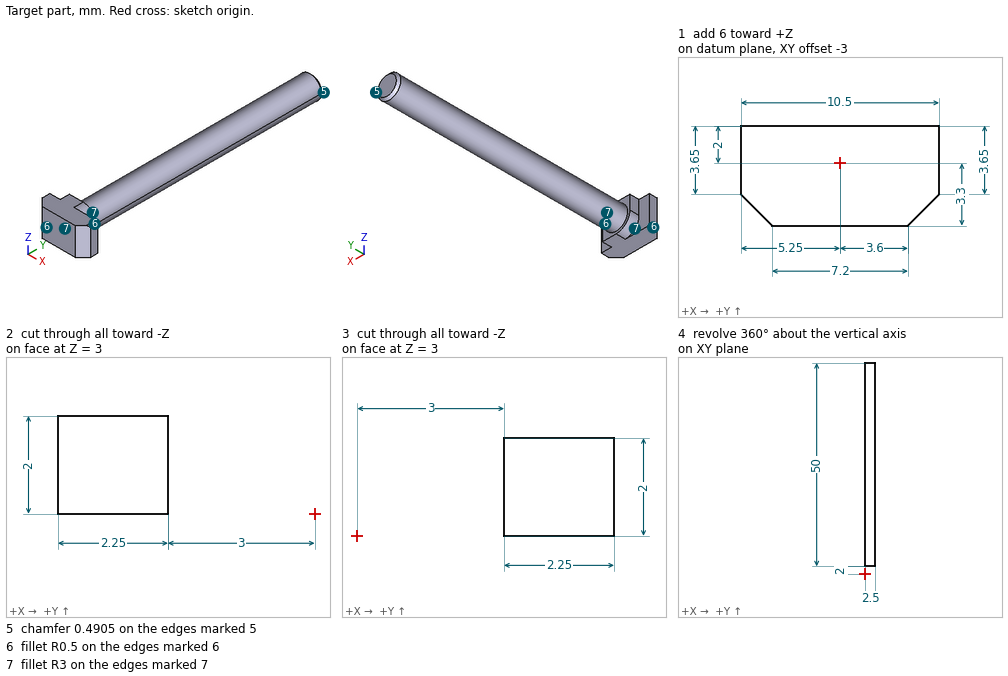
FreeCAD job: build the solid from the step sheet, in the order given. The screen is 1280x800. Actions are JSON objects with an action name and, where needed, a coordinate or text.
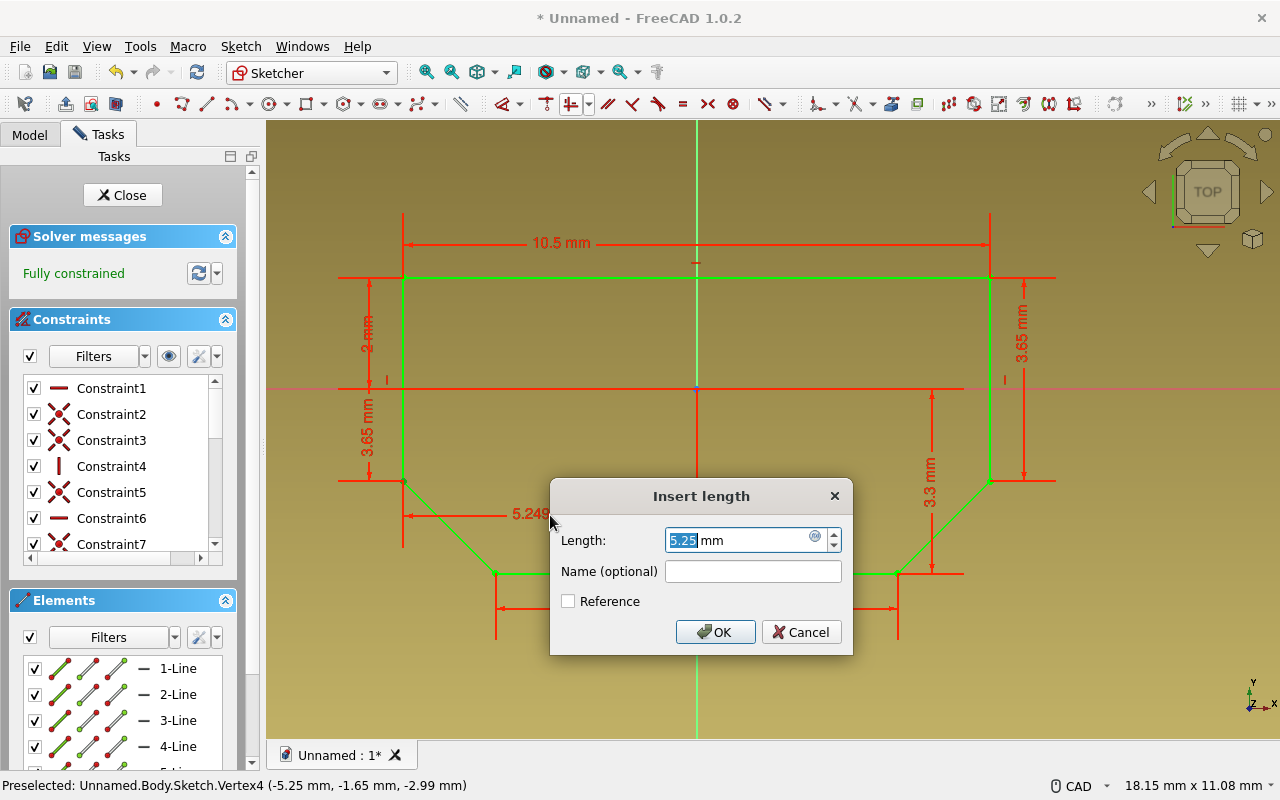
{"action": "type", "text": "5.25"}
{"action": "key", "text": "Return"}
{"action": "key", "text": "Escape"}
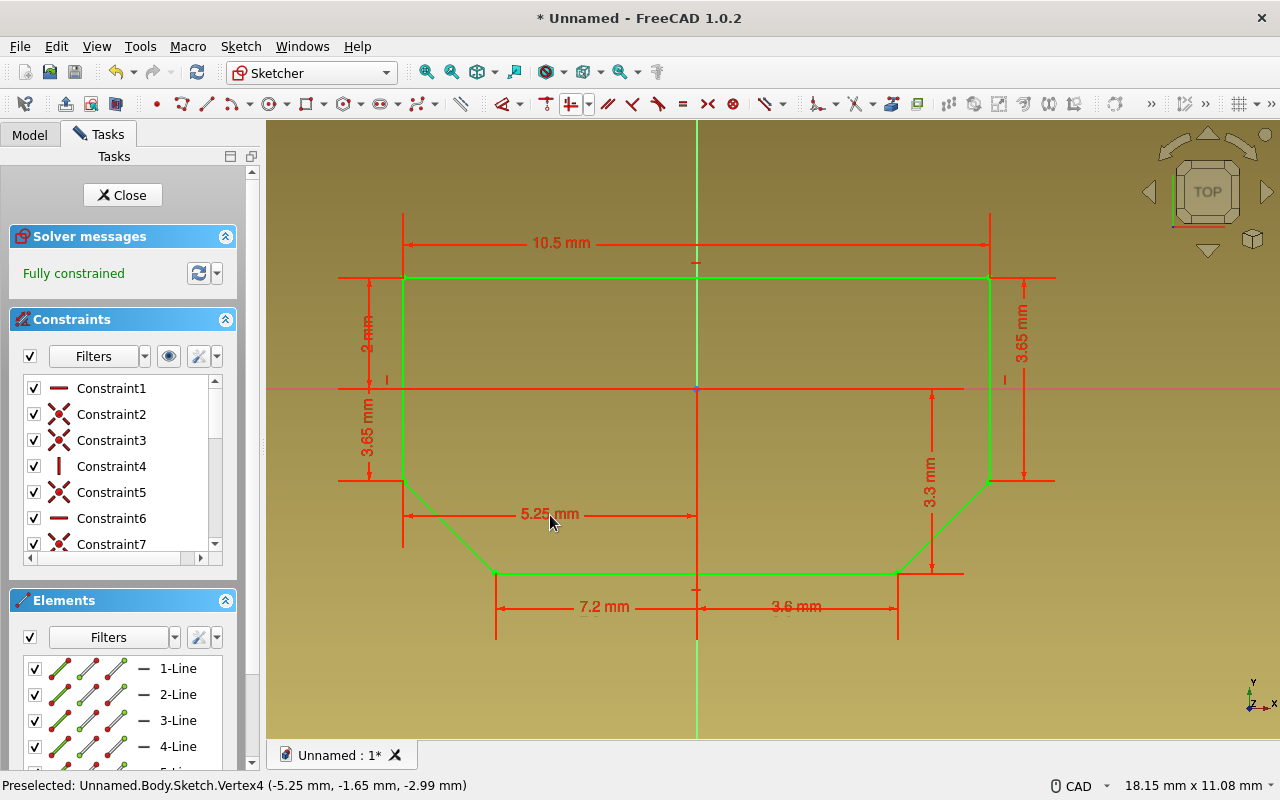
{"action": "left_click", "coordinate": [123, 195]}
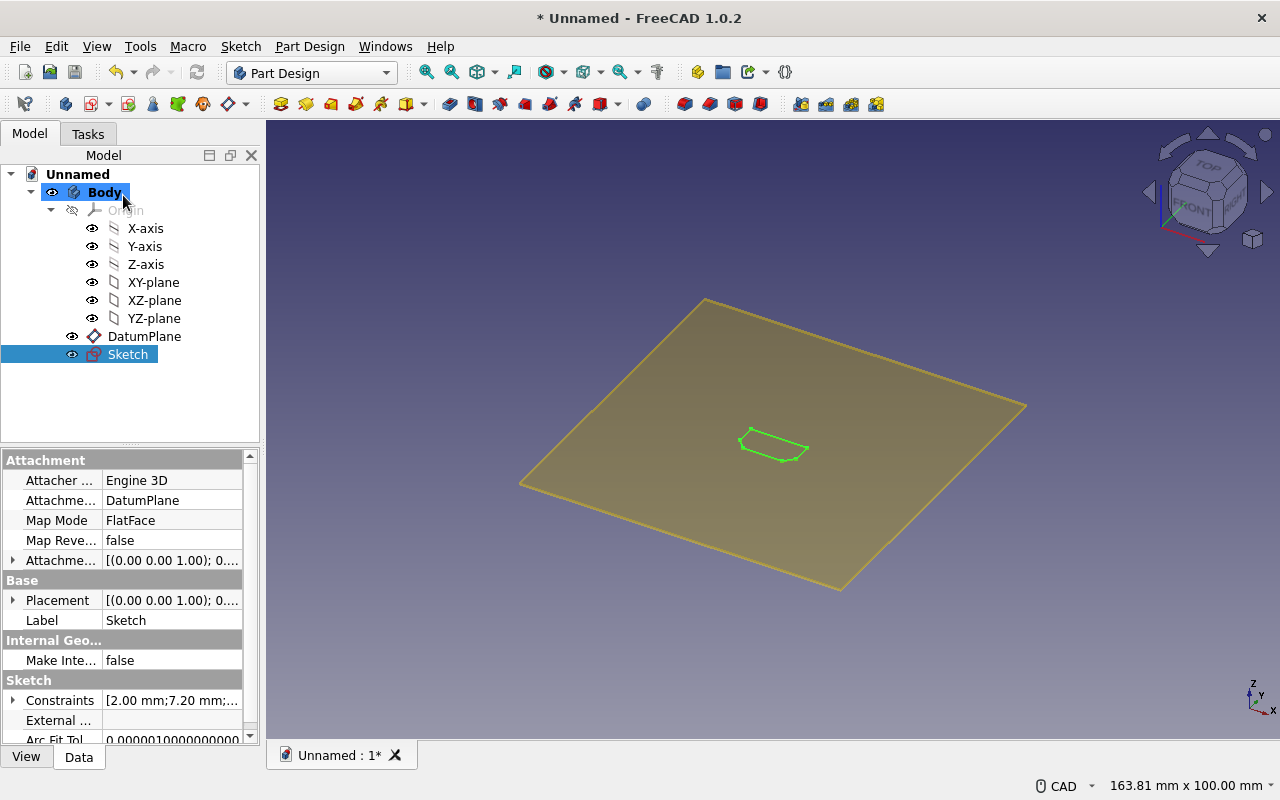
{"action": "left_click", "coordinate": [281, 104]}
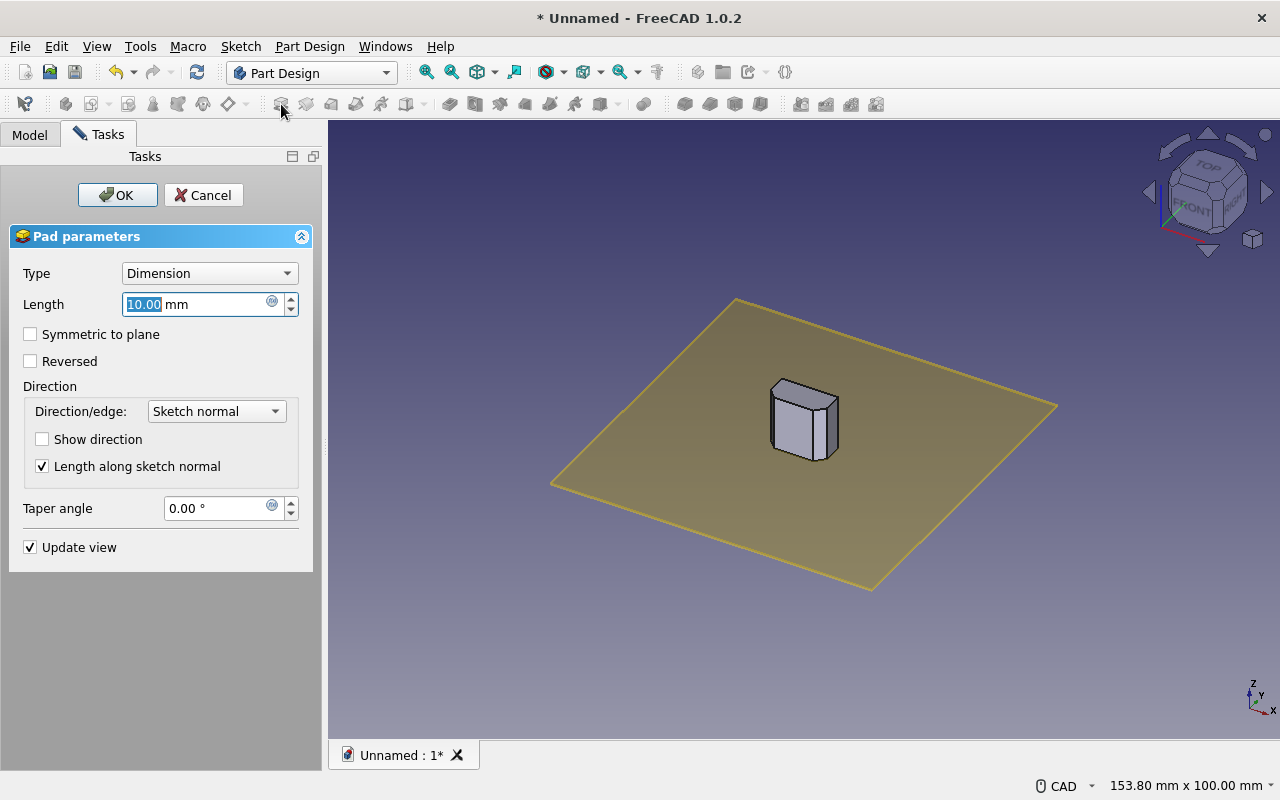
{"action": "type", "text": "6"}
{"action": "key", "text": "Tab"}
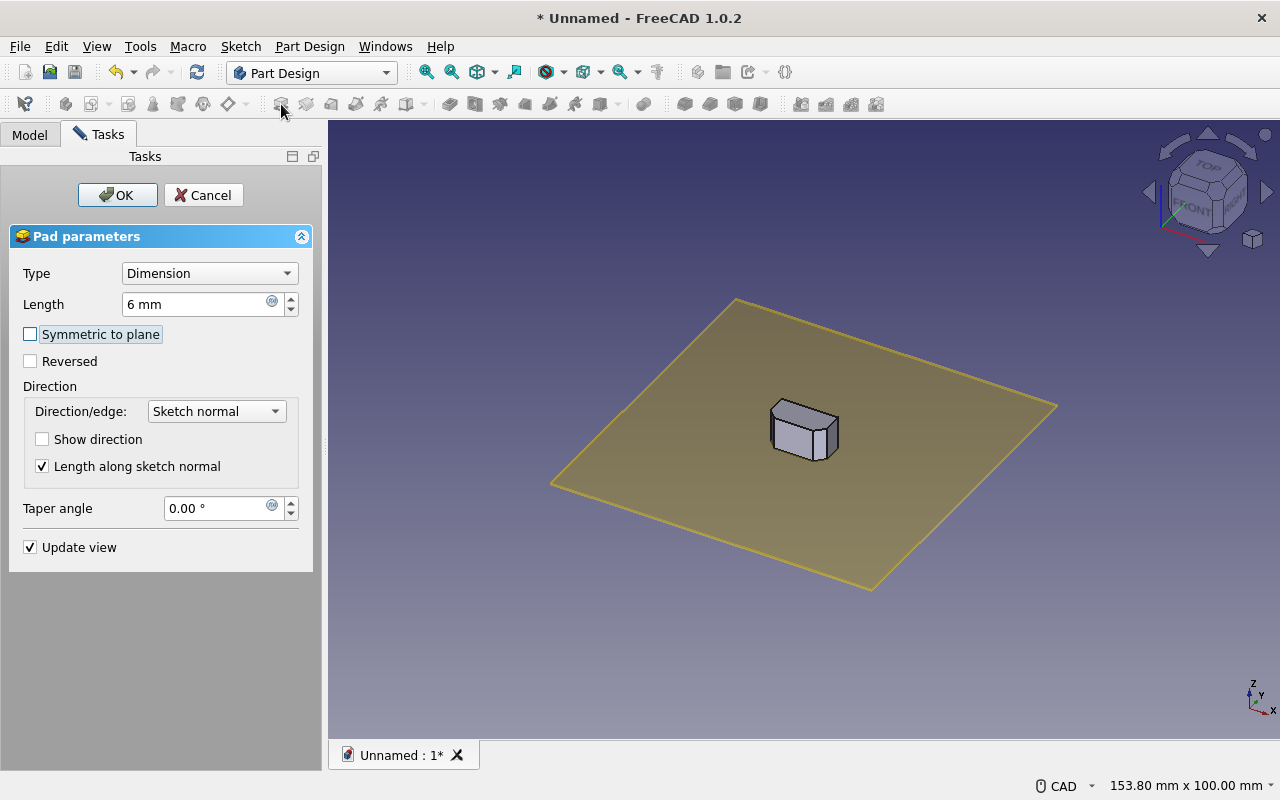
{"action": "left_click", "coordinate": [118, 195]}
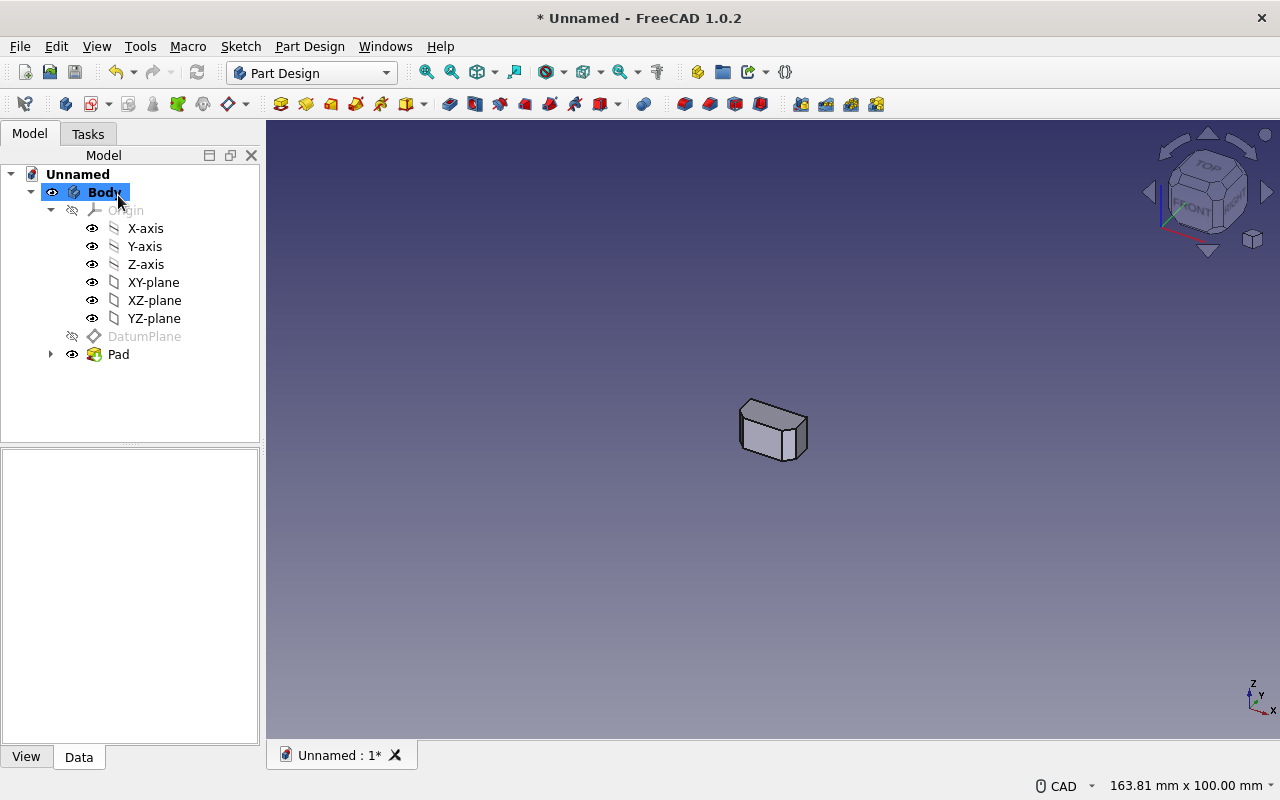
{"action": "left_click", "coordinate": [427, 72]}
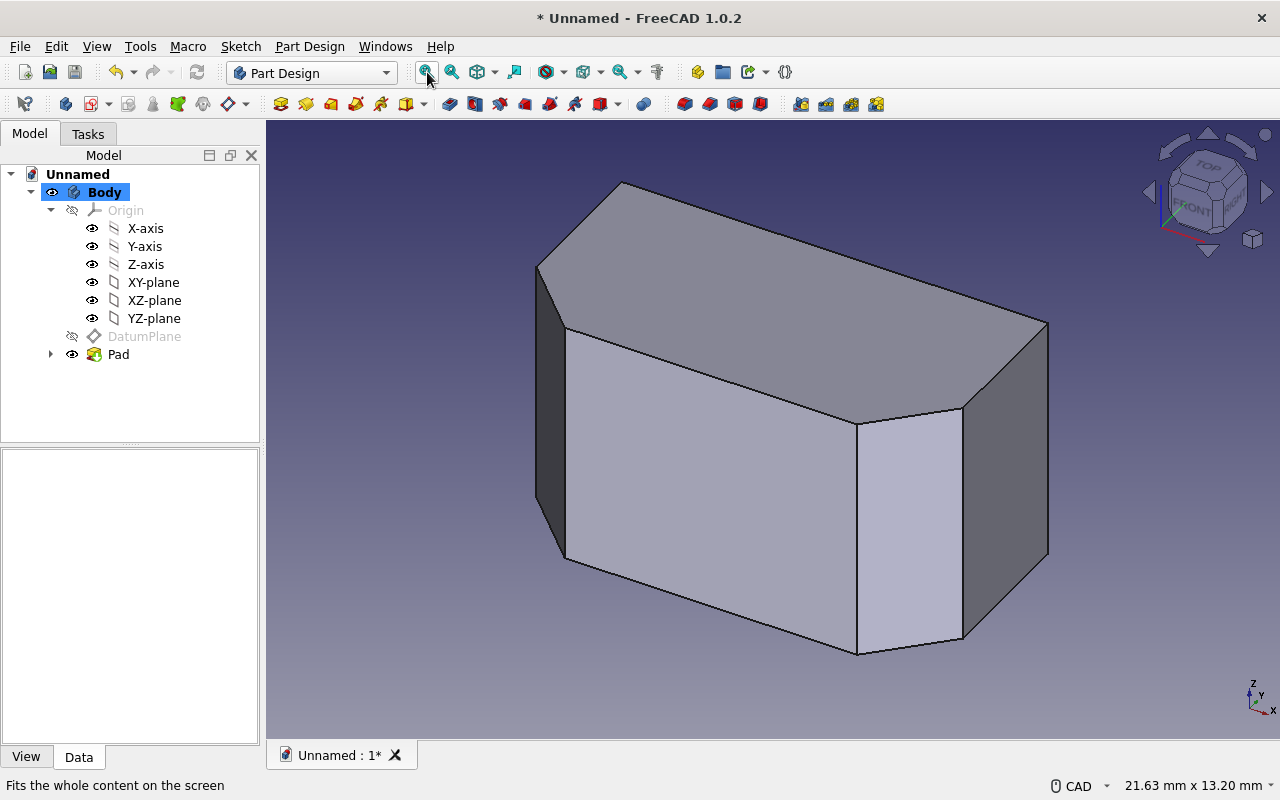
{"action": "left_click", "coordinate": [834, 333]}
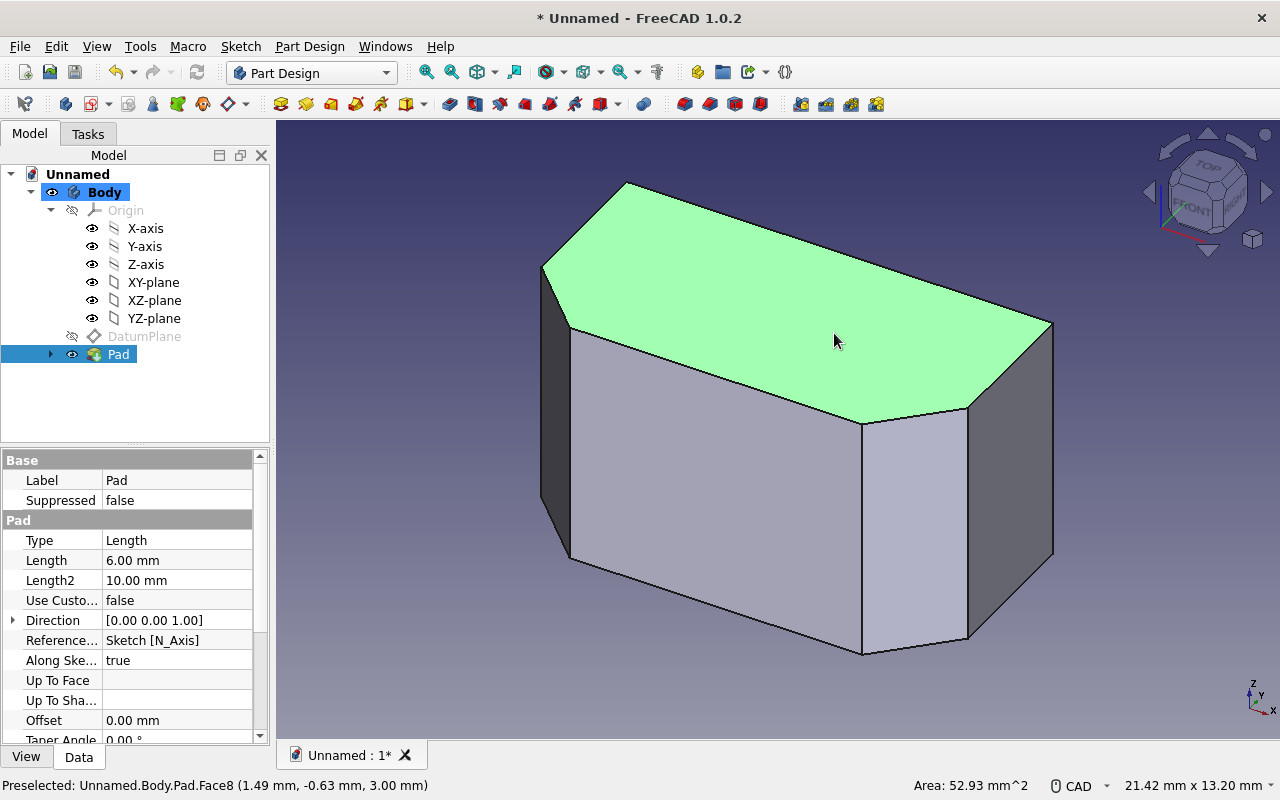
{"action": "left_click", "coordinate": [90, 104]}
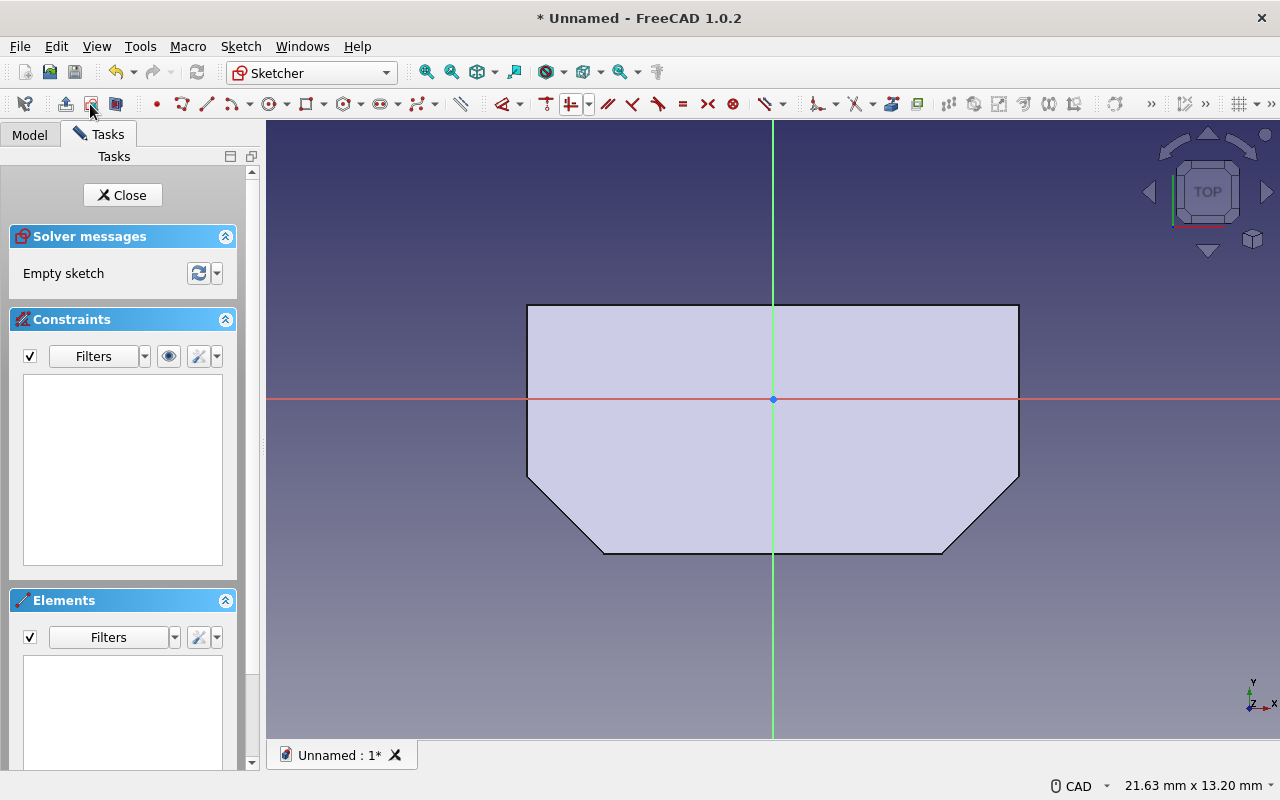
{"action": "scroll", "coordinate": [605, 289], "scroll_direction": "up", "scroll_amount": 4}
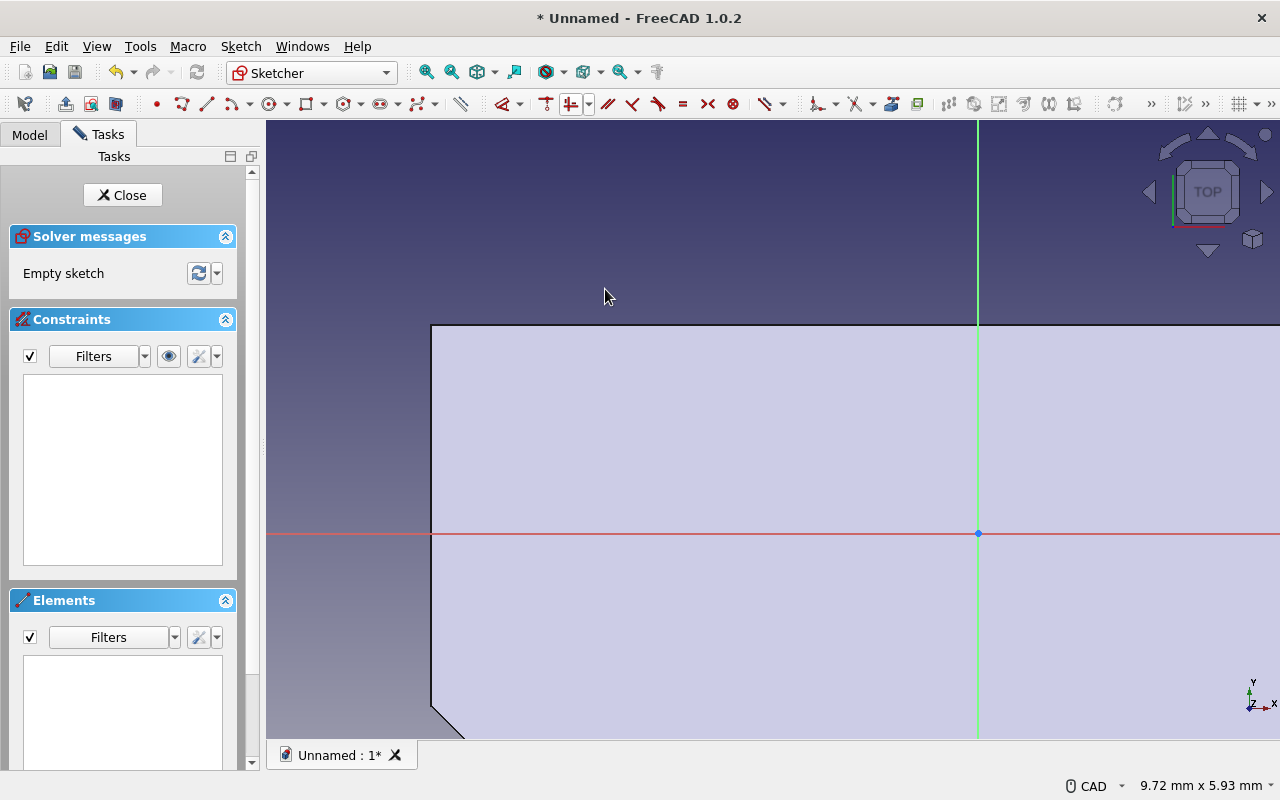
{"action": "key", "text": "g r"}